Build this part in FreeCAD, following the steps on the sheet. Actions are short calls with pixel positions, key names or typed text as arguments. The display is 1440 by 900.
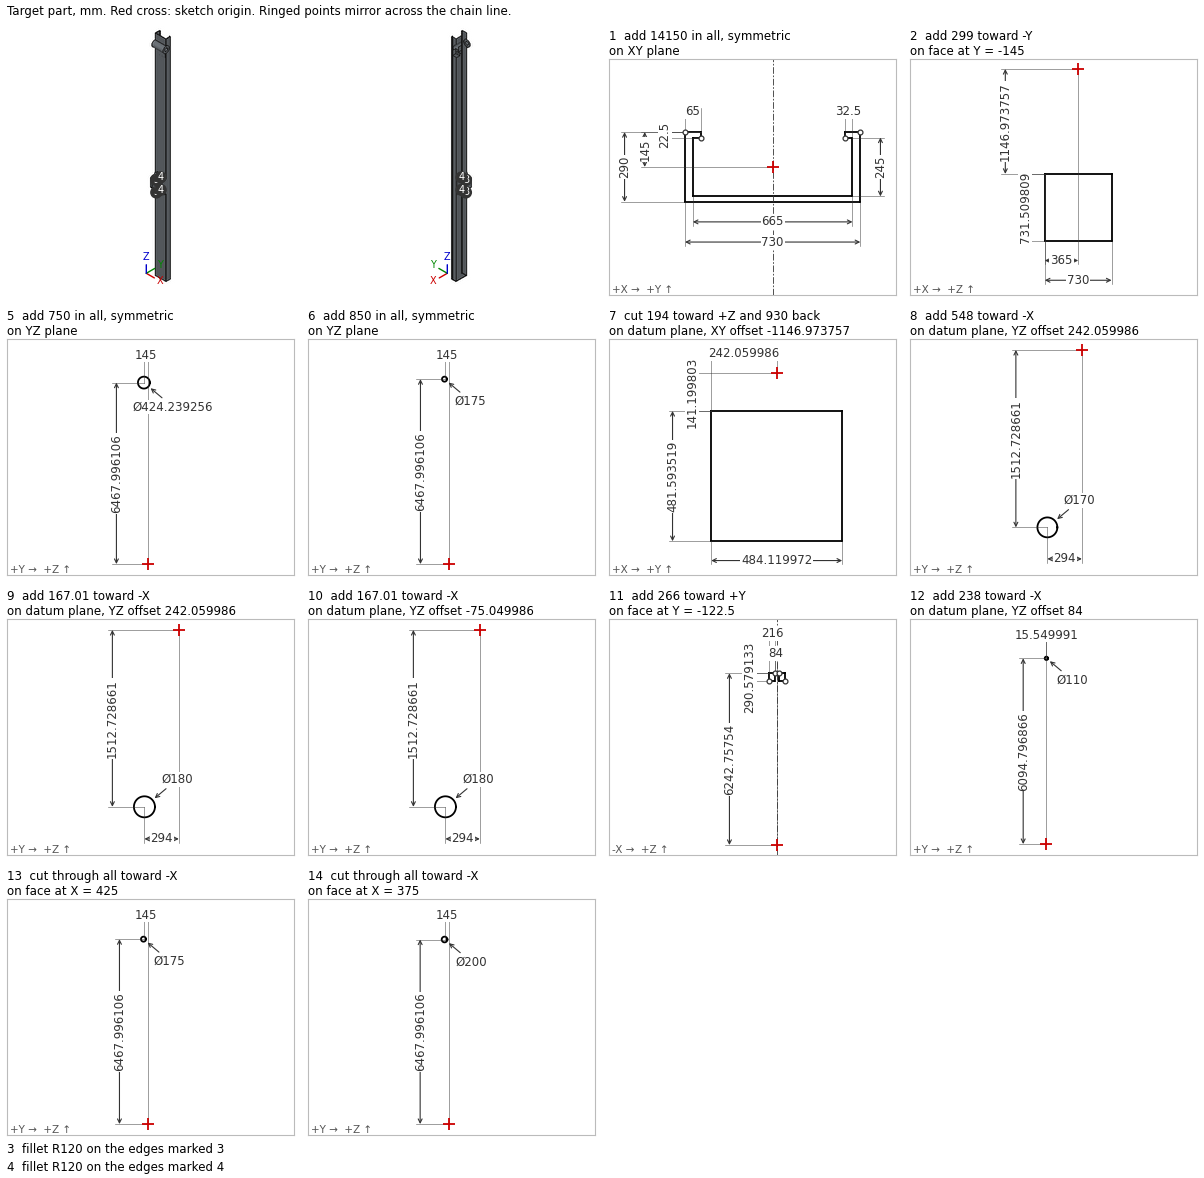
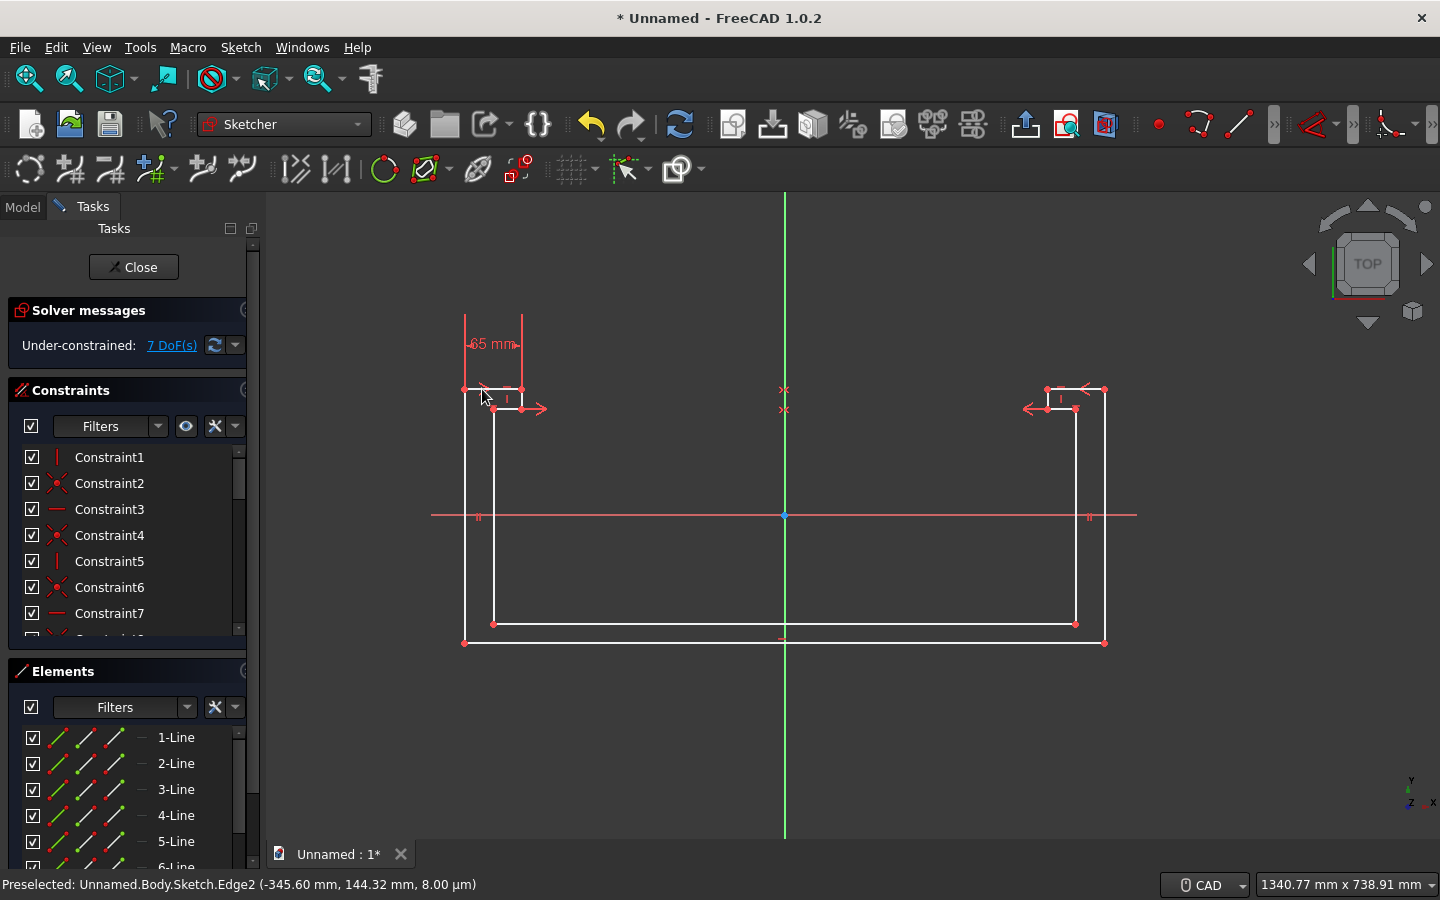
click(465, 465)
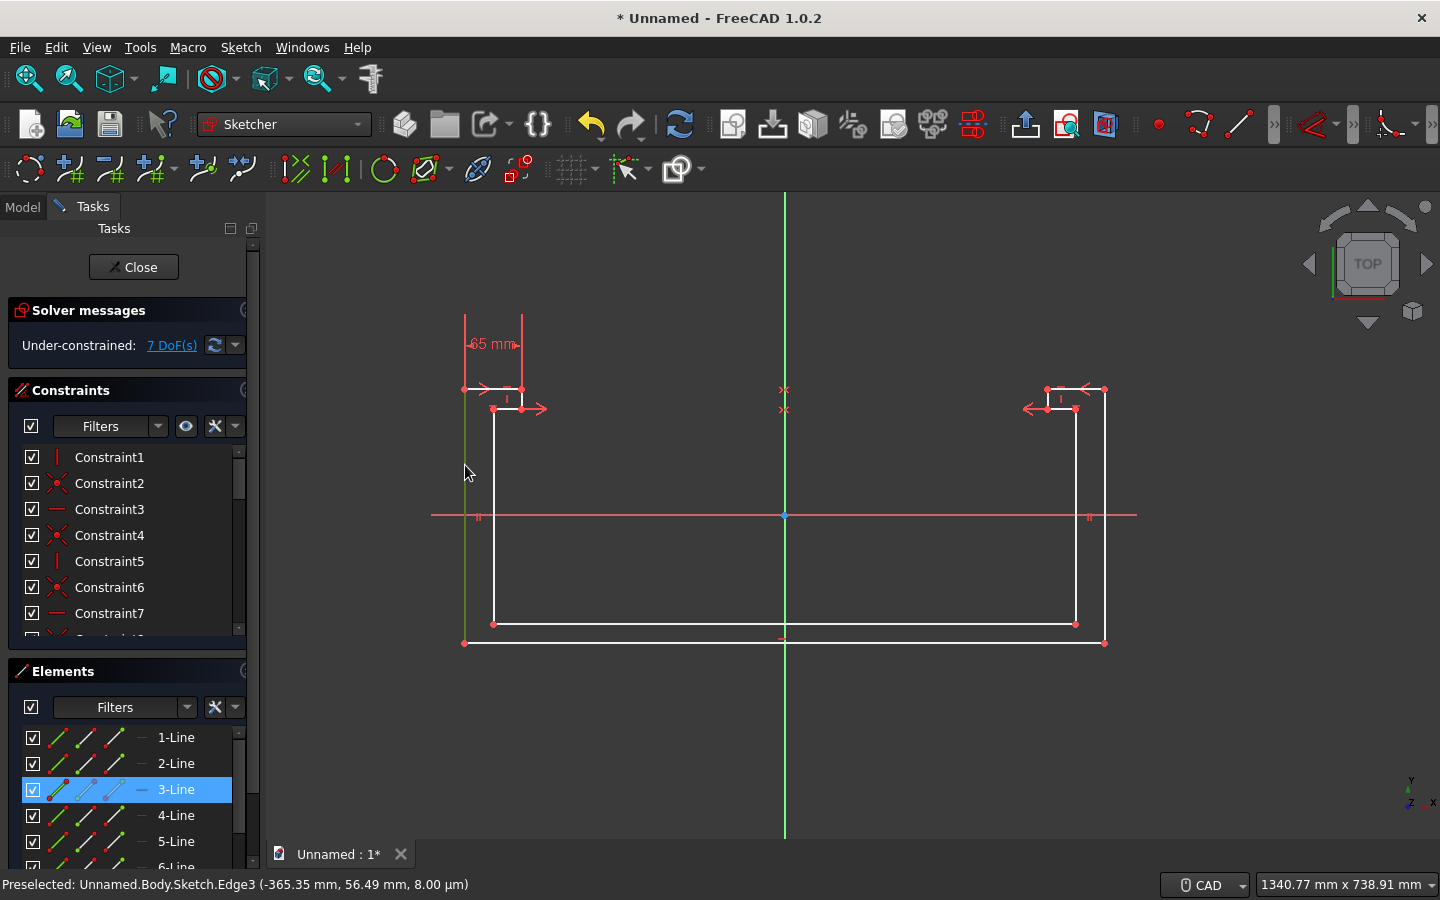
click(1338, 124)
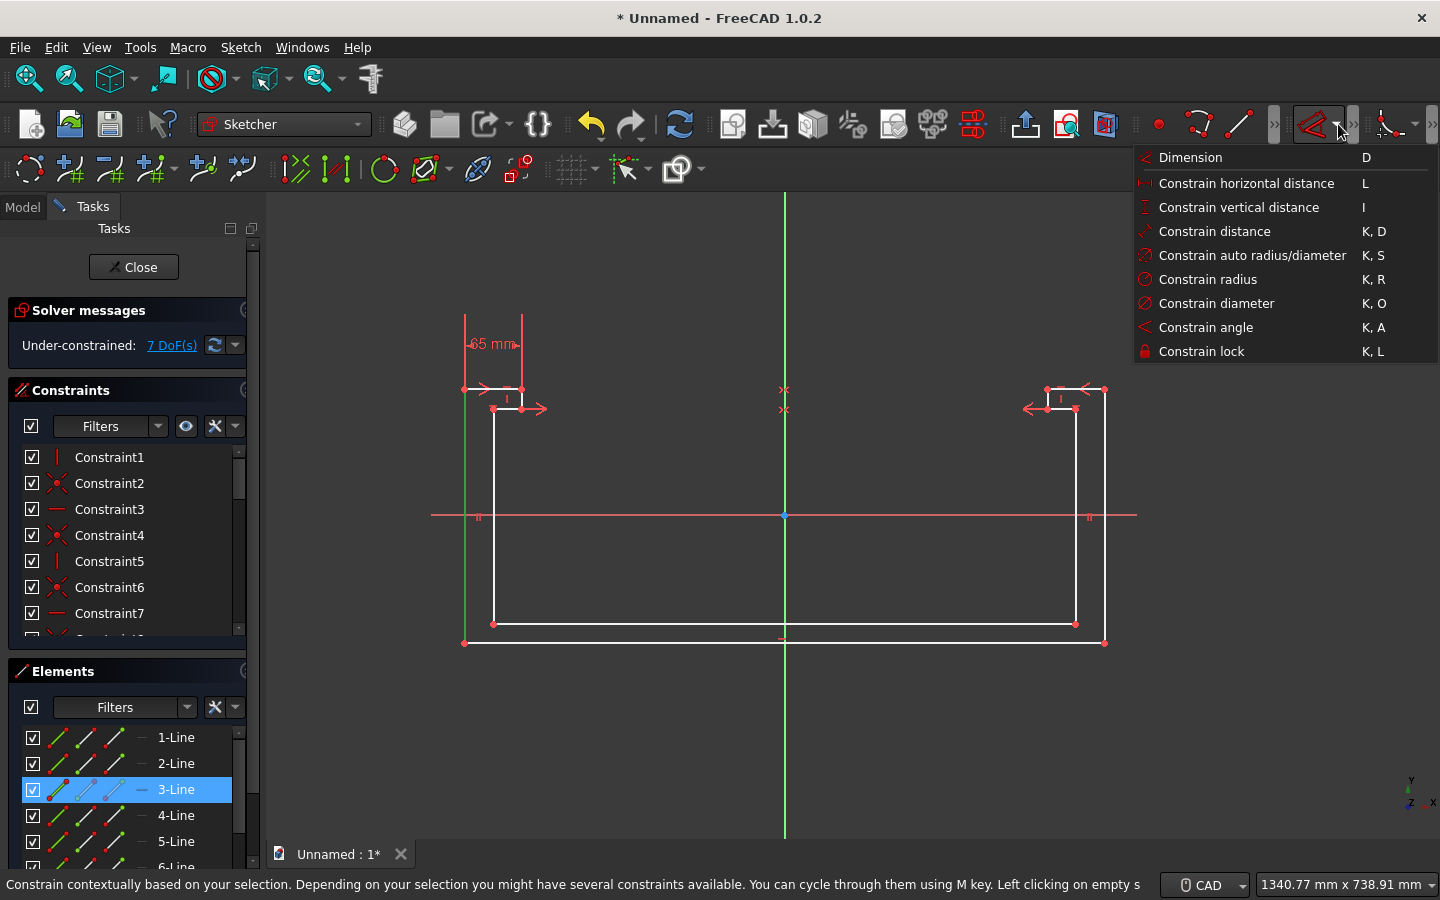
click(1286, 207)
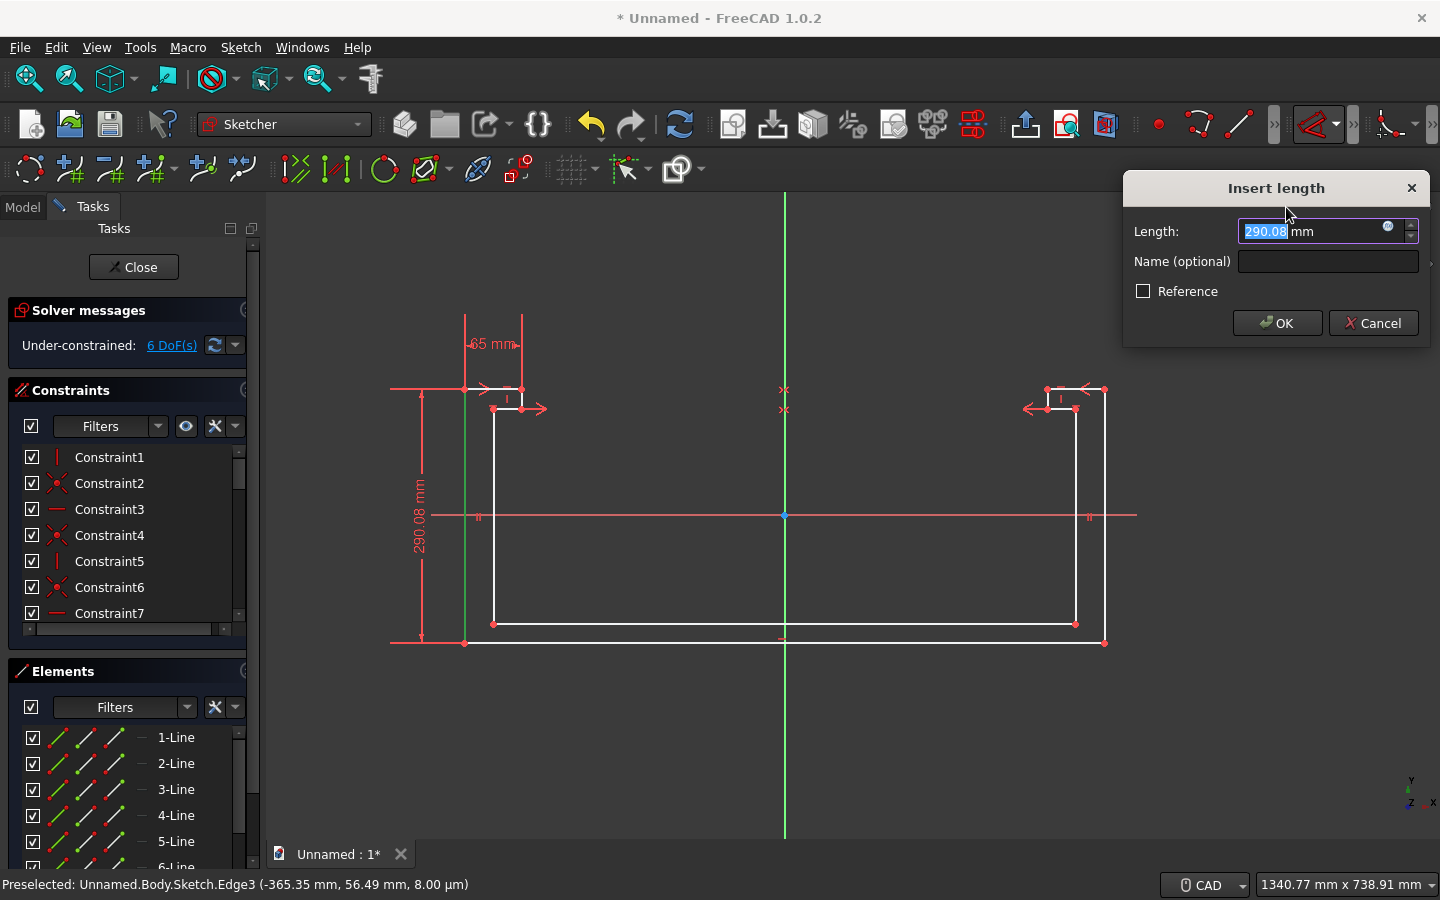
text(290)
key(Return)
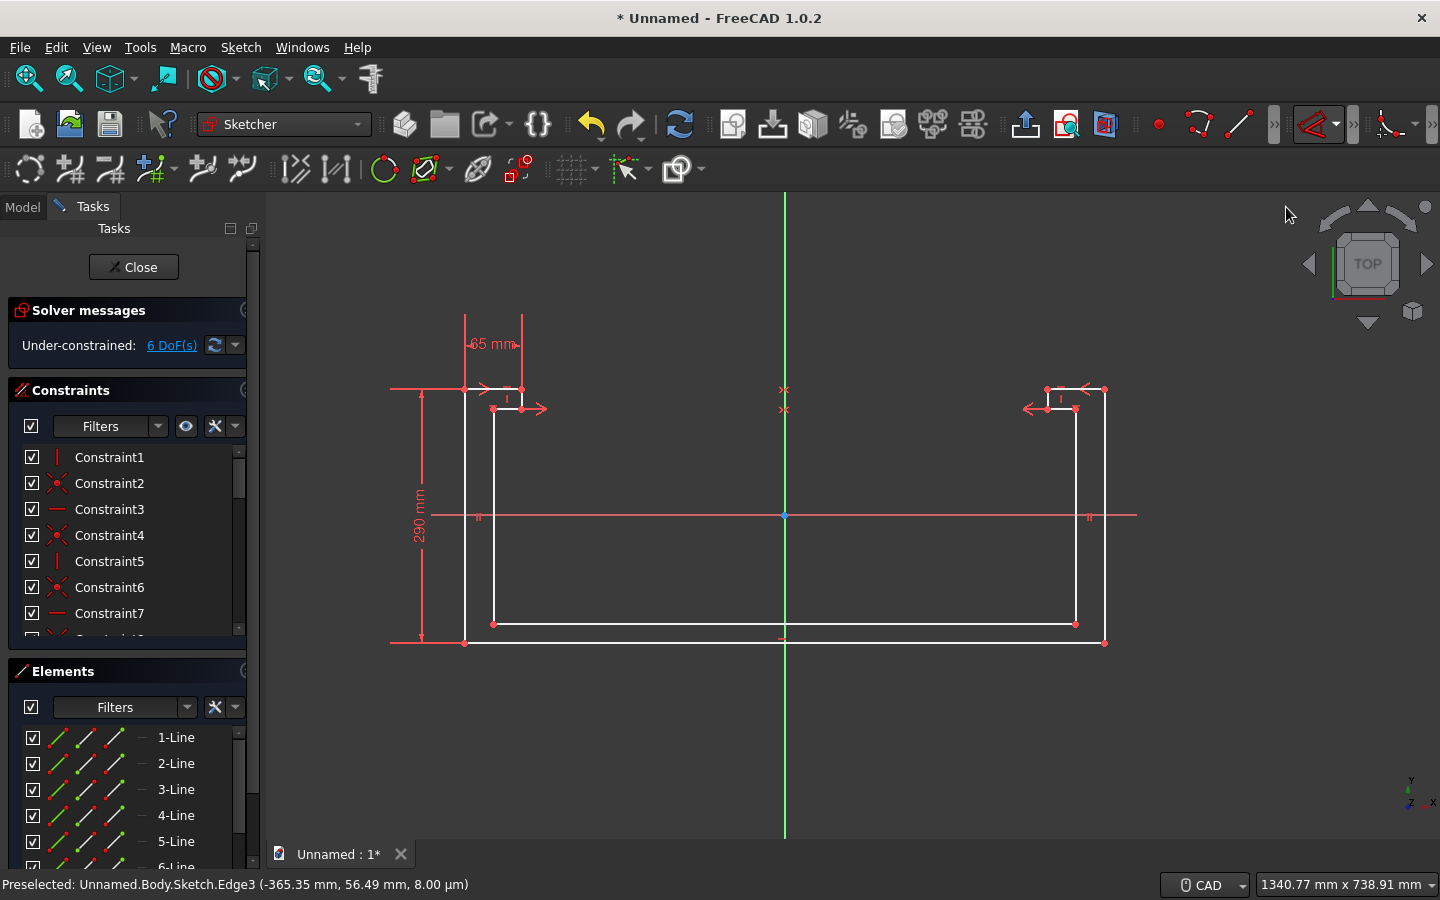
click(657, 643)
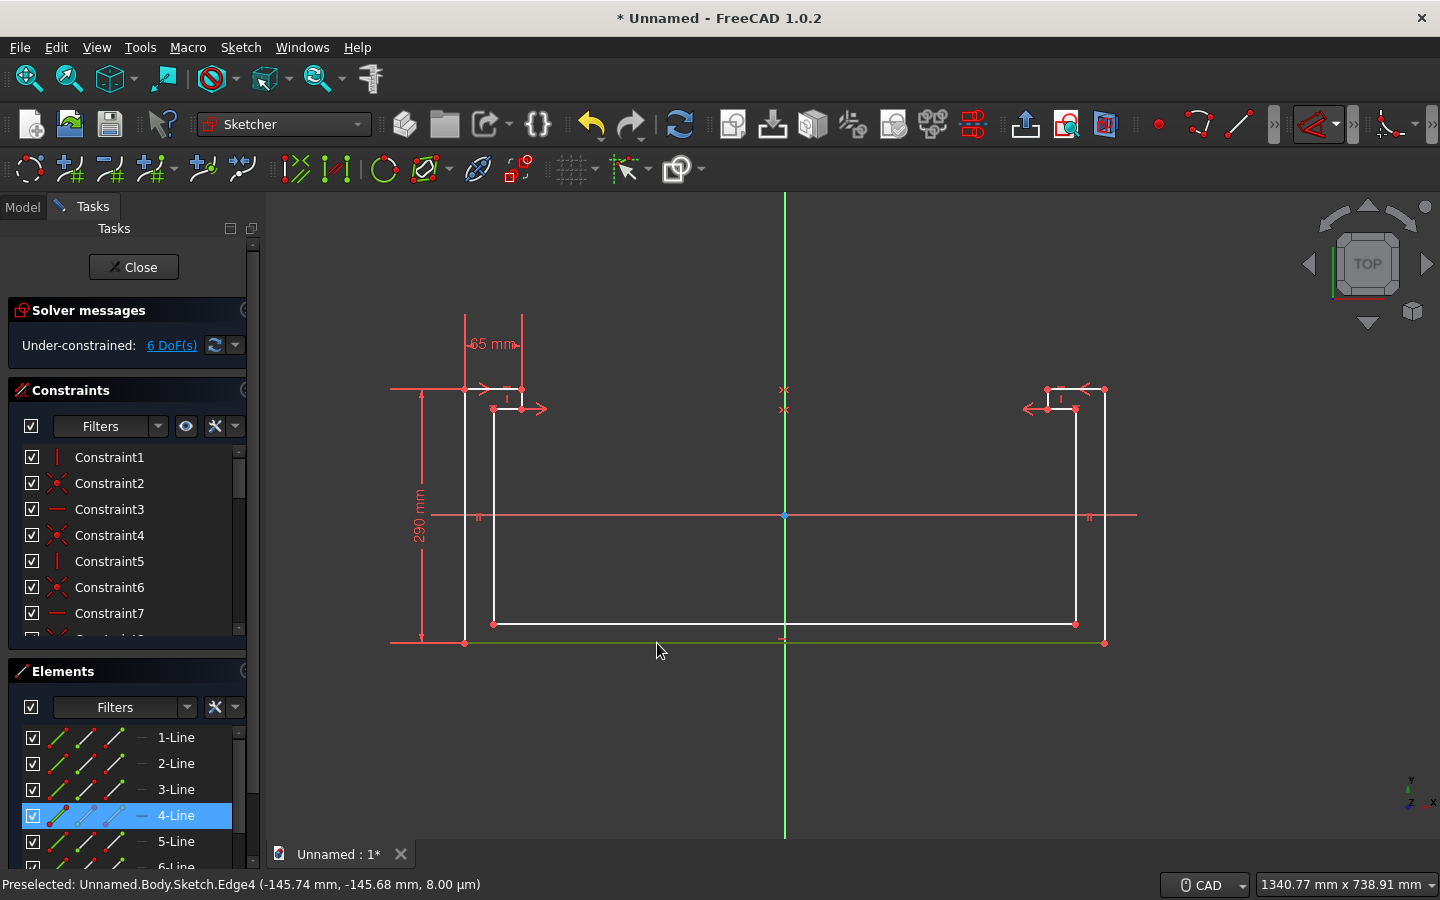
key(l)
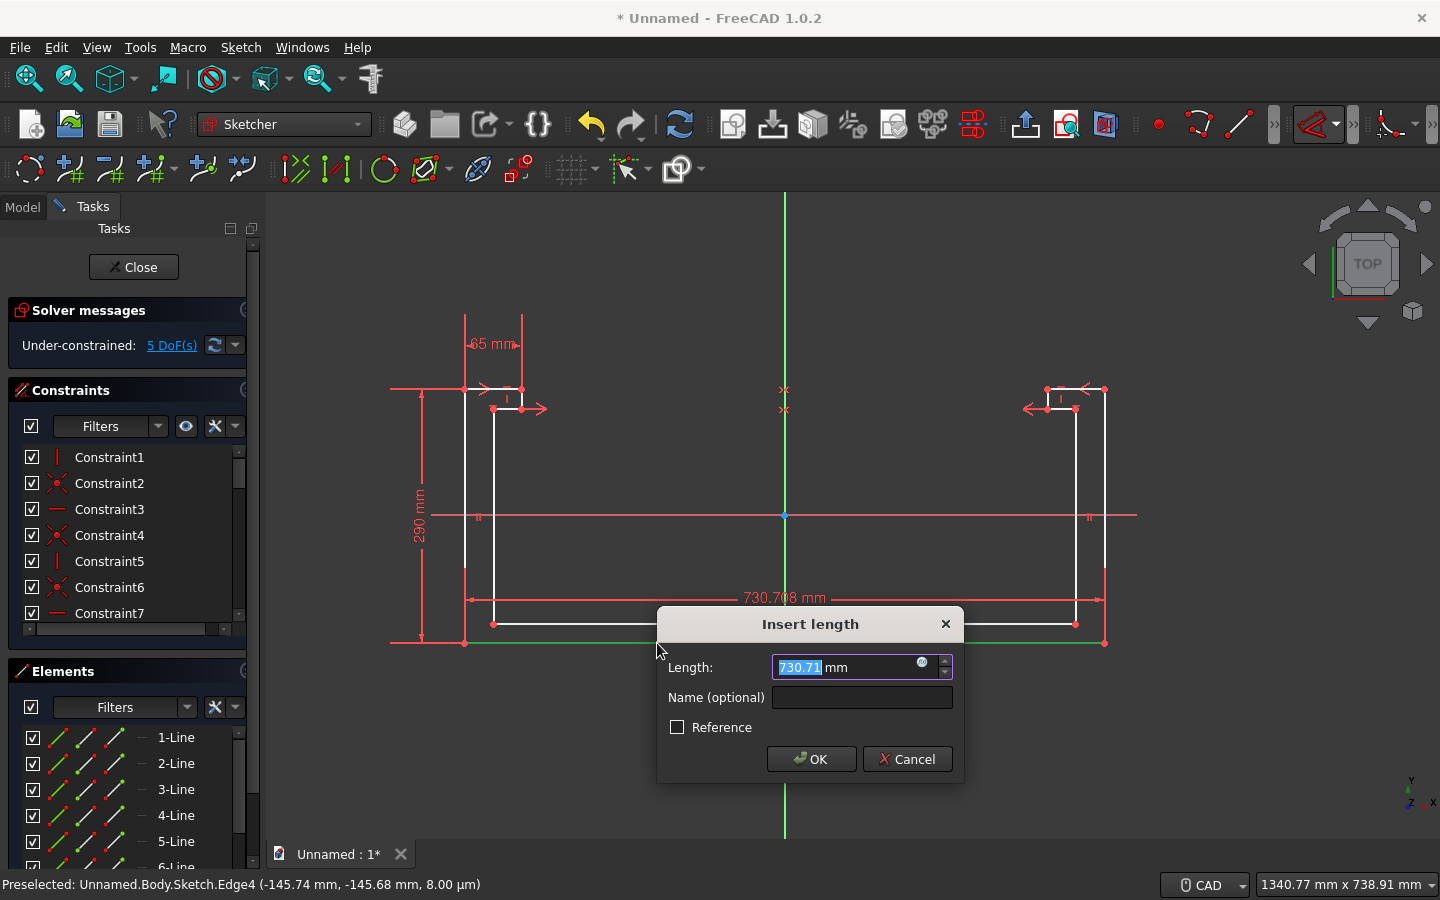
text(730)
key(Return)